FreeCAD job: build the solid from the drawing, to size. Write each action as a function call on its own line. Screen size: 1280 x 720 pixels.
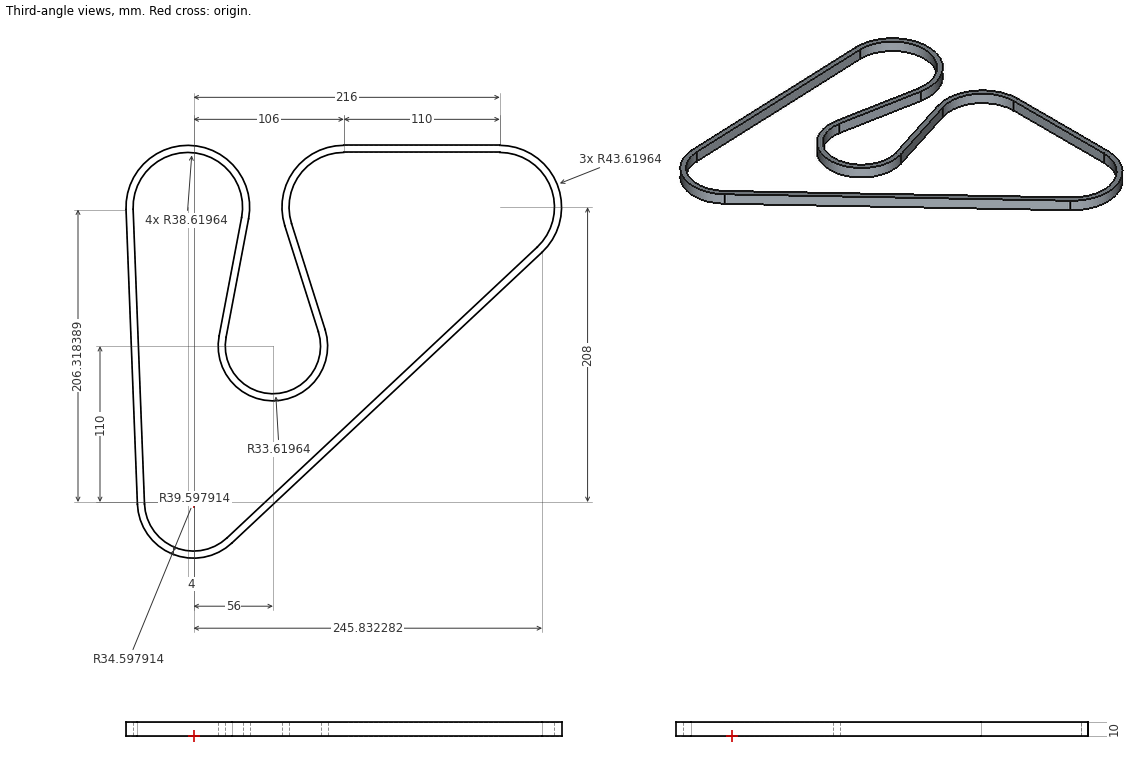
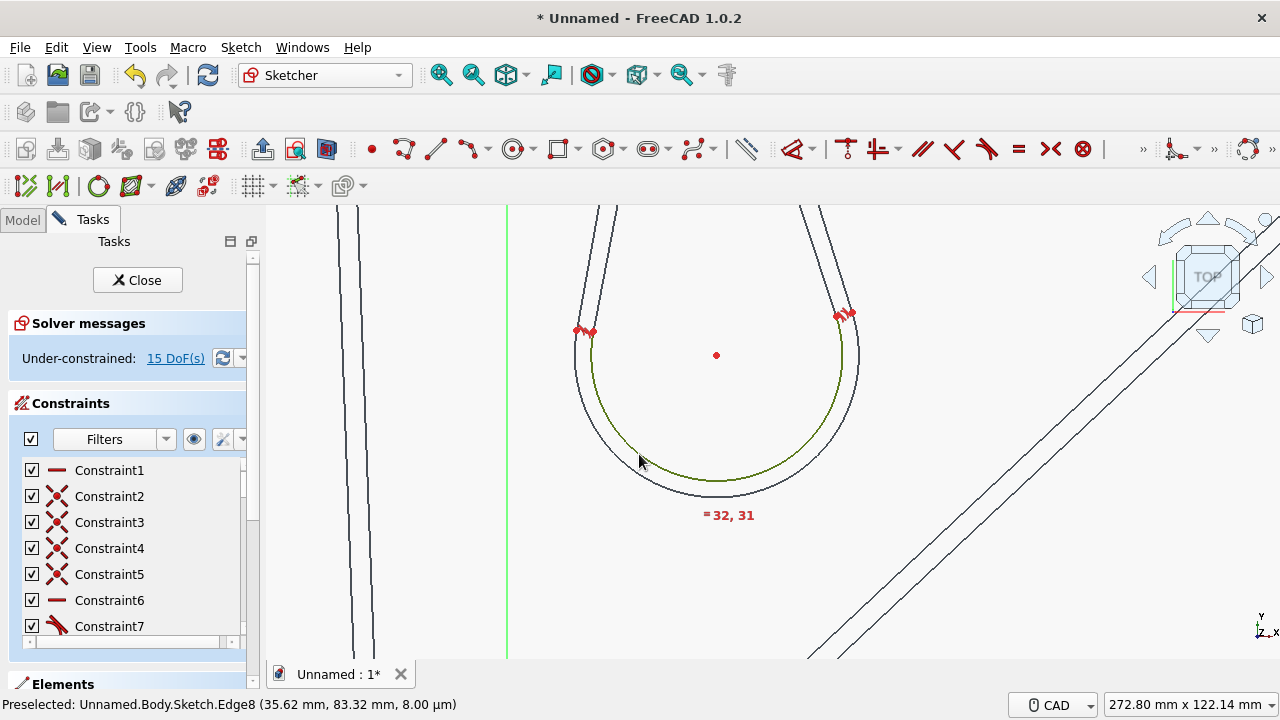
key(k)
key(r)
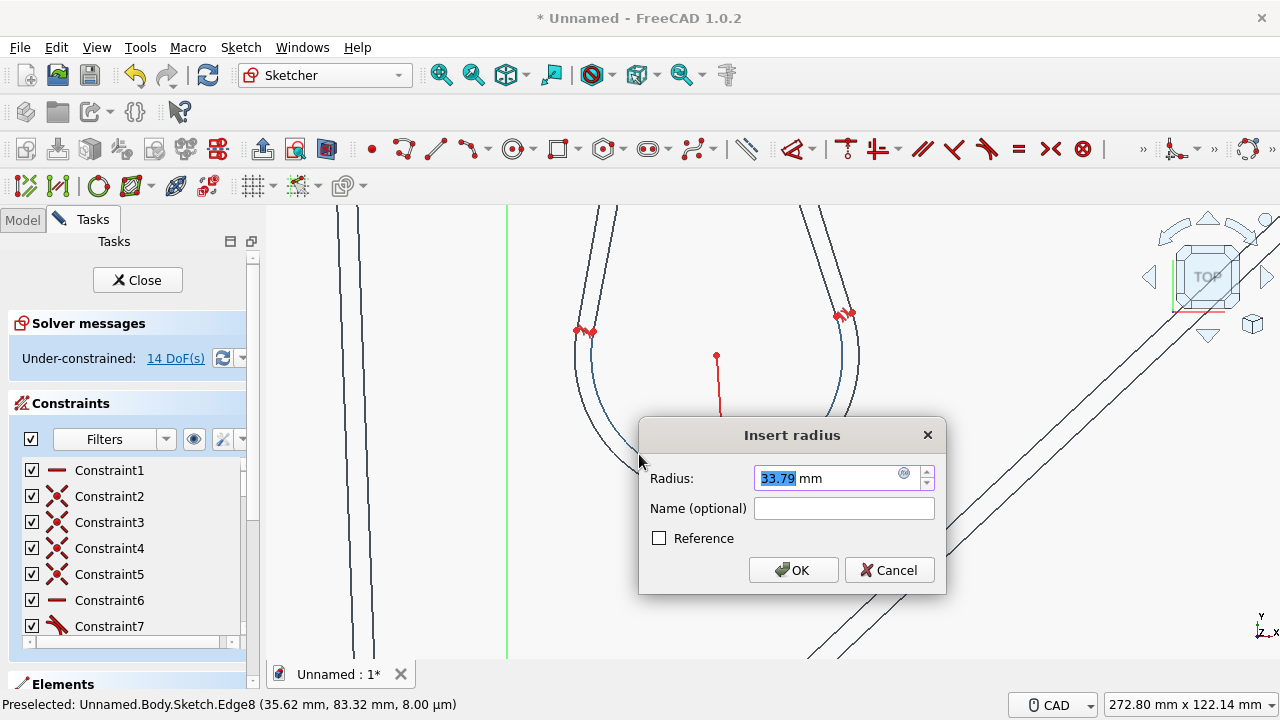
text(33.61964)
key(Return)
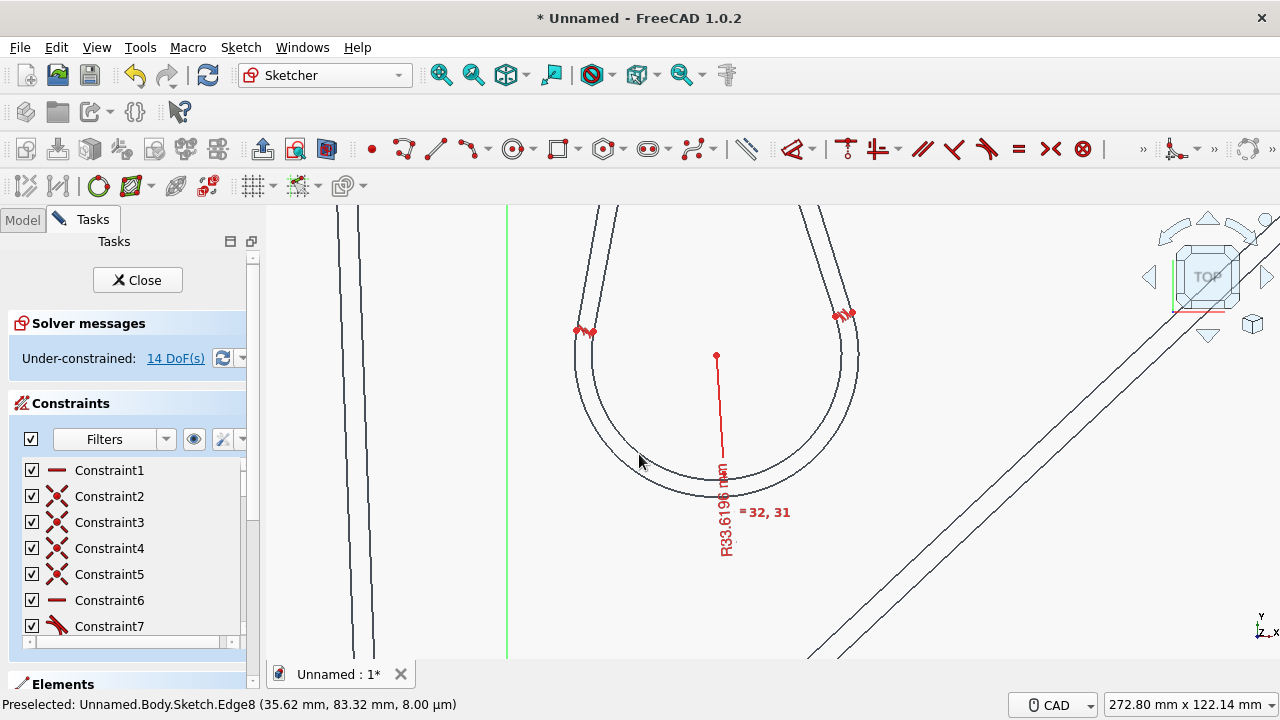
scroll(642, 454, down, 7)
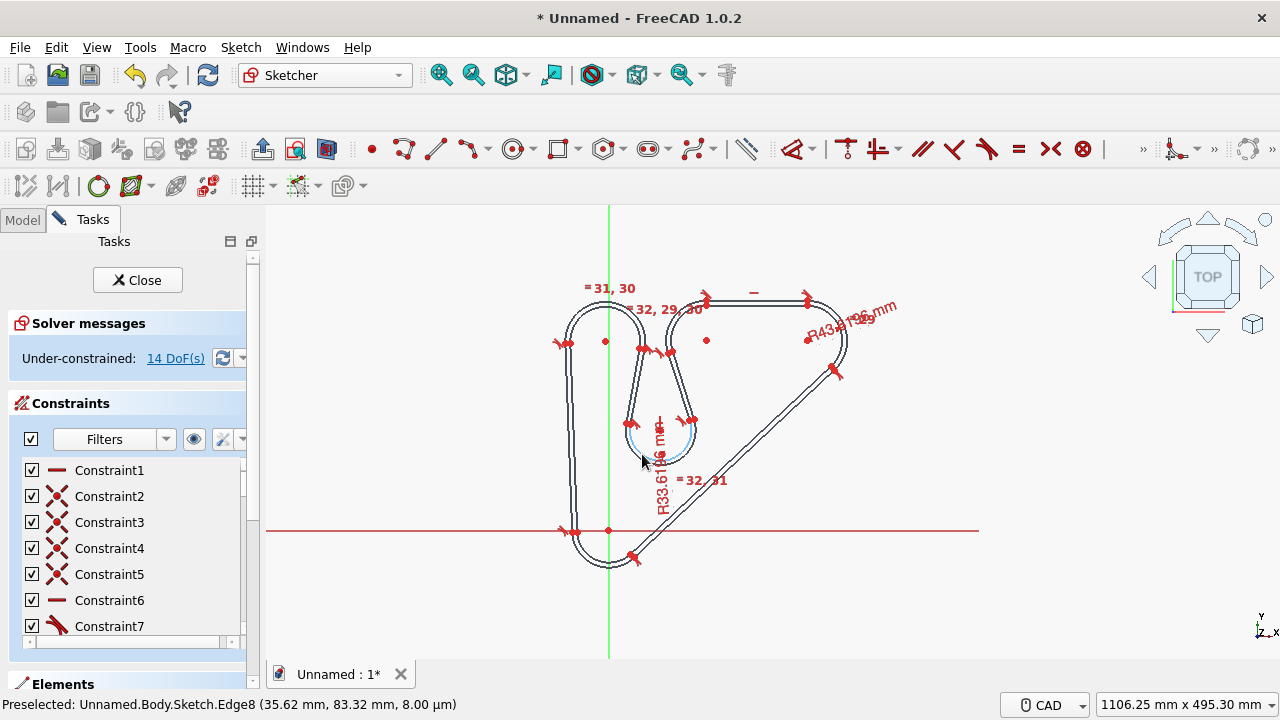
scroll(581, 555, up, 6)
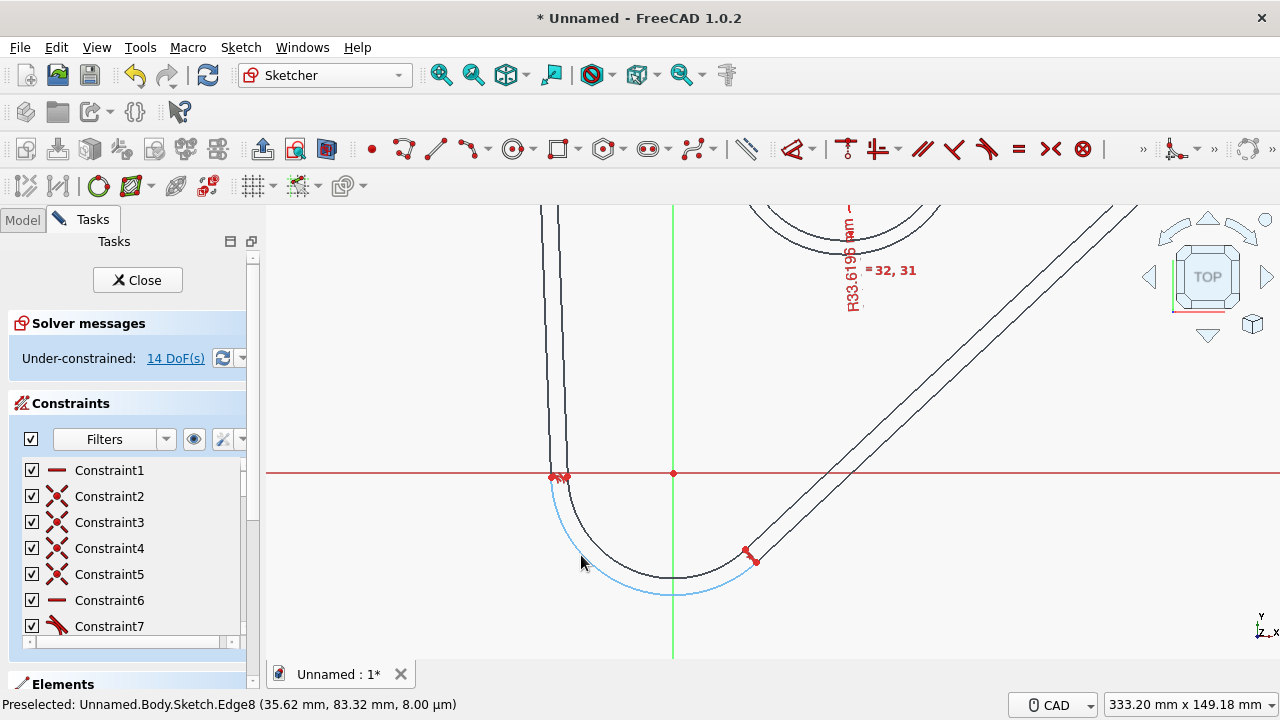
click(582, 554)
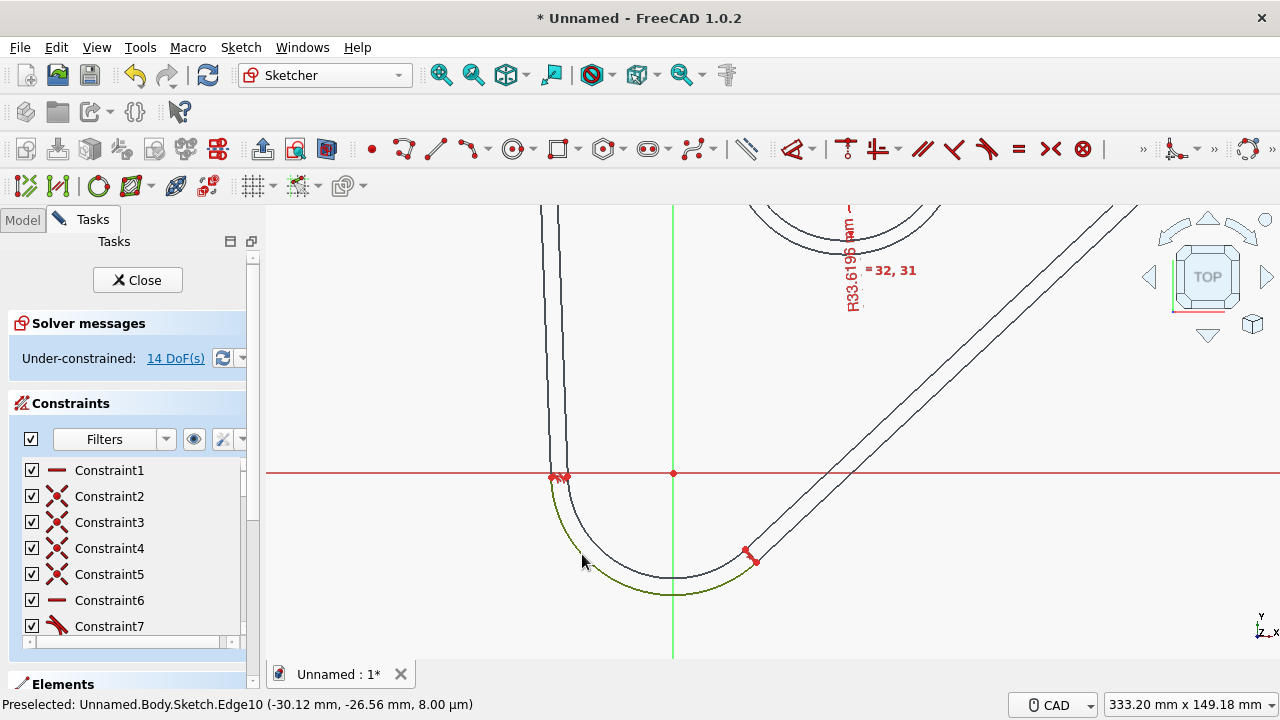
click(814, 150)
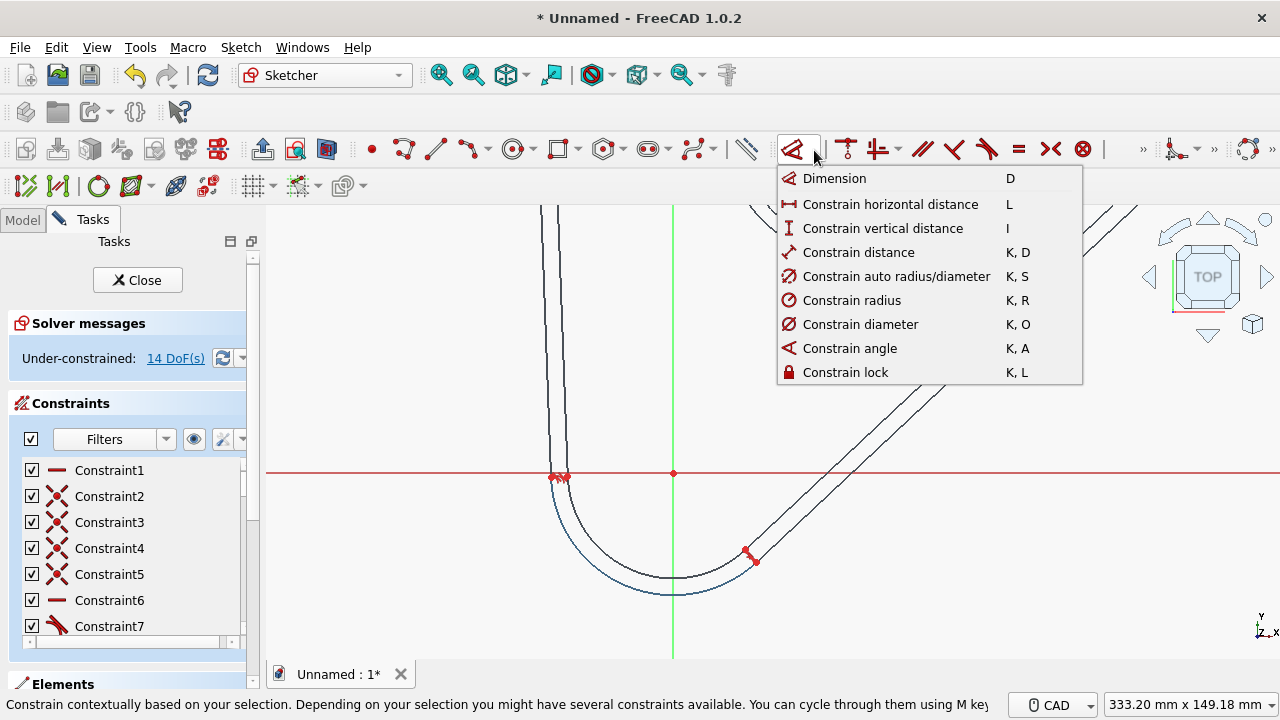
click(930, 300)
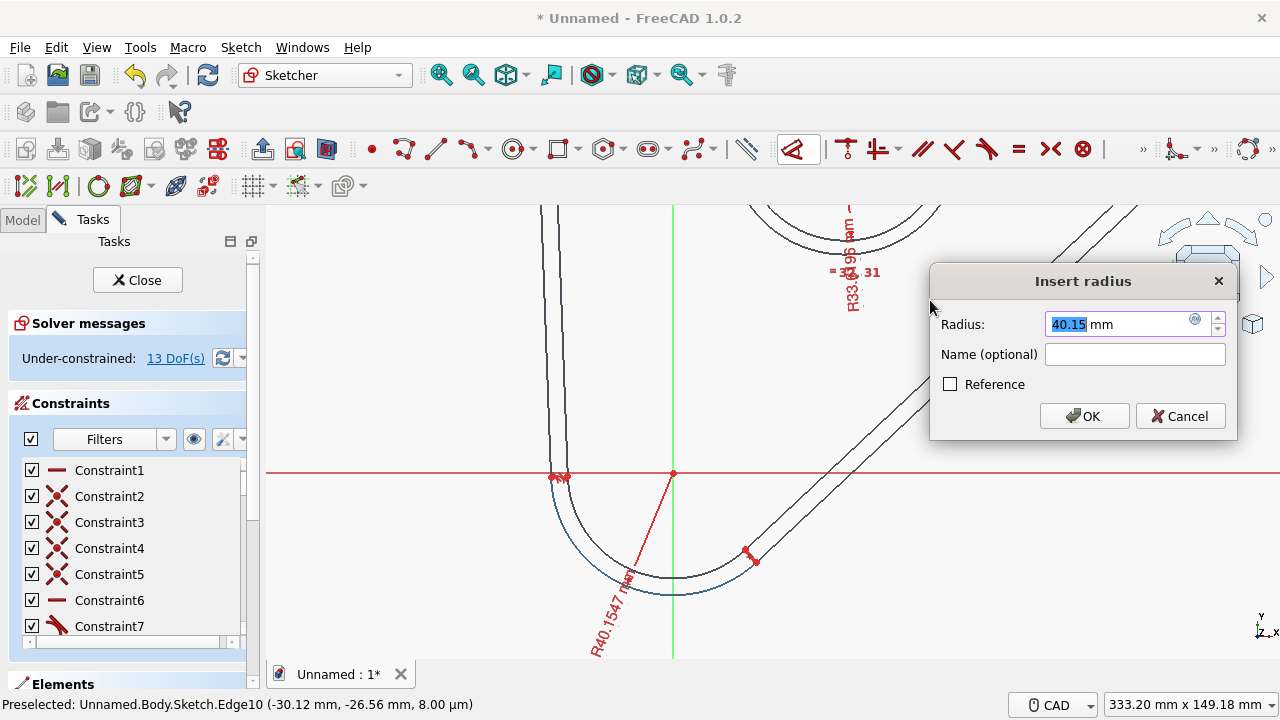
text(39.597914)
key(Return)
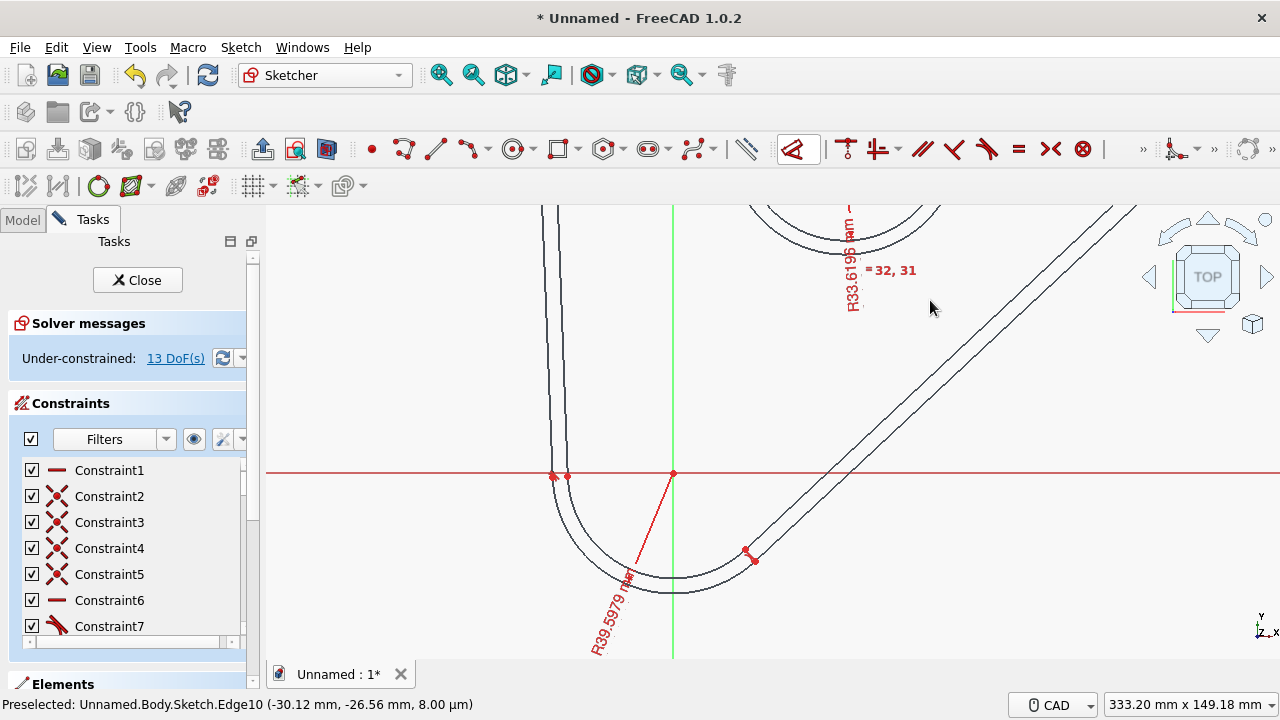
click(594, 543)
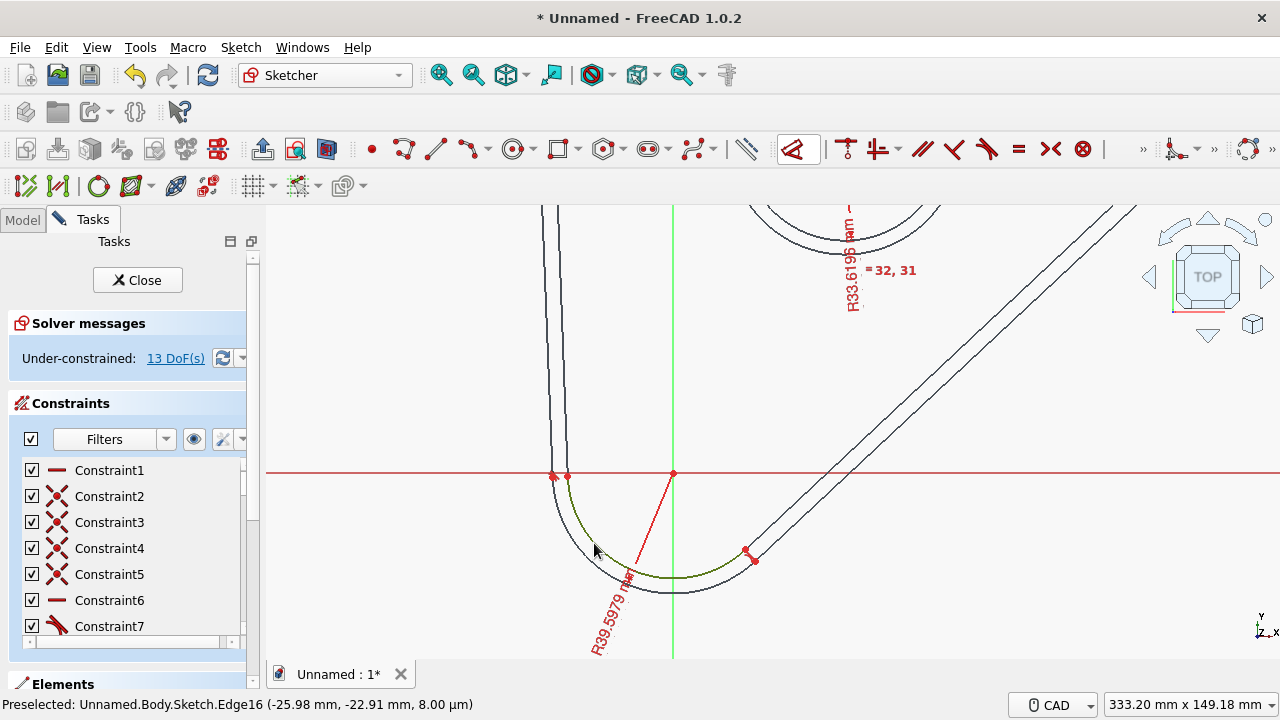
key(k)
key(r)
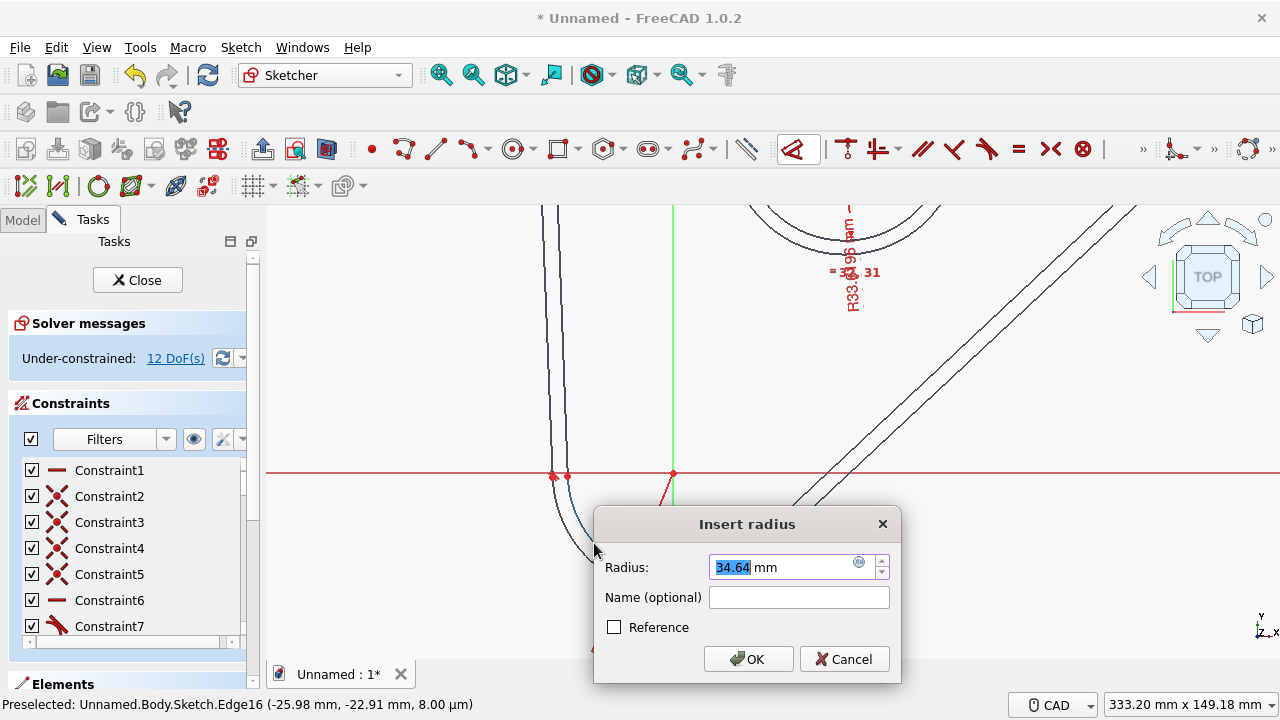
text(34.597914)
key(Return)